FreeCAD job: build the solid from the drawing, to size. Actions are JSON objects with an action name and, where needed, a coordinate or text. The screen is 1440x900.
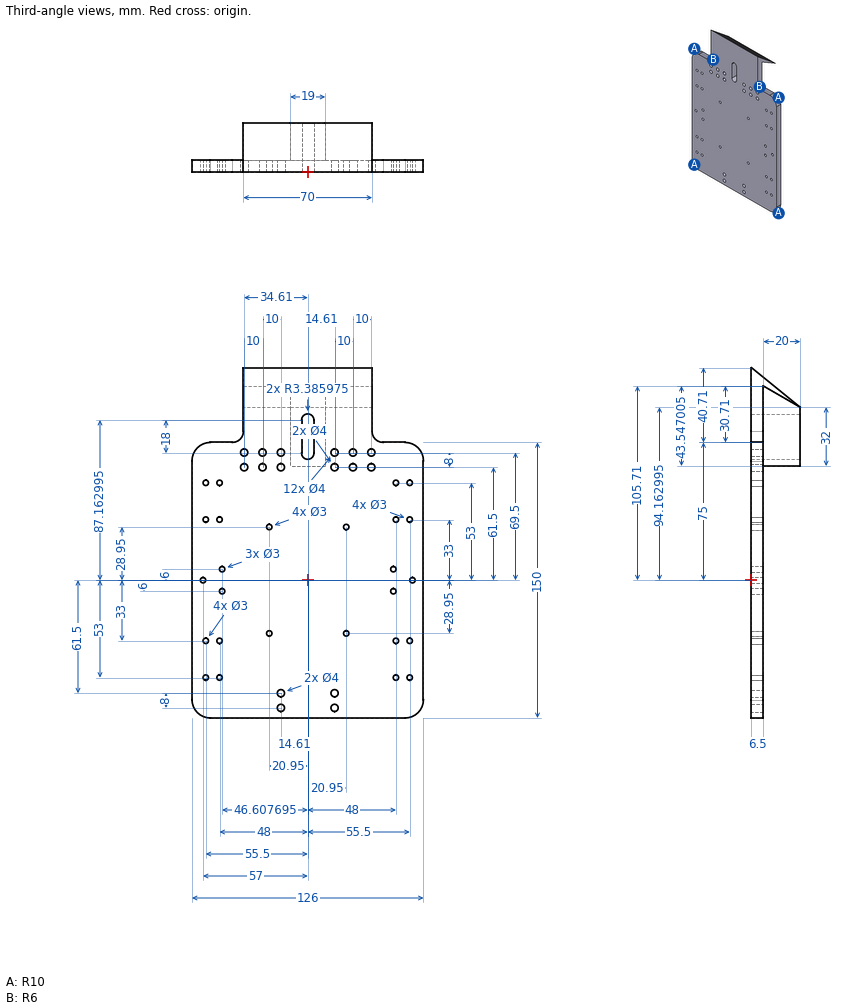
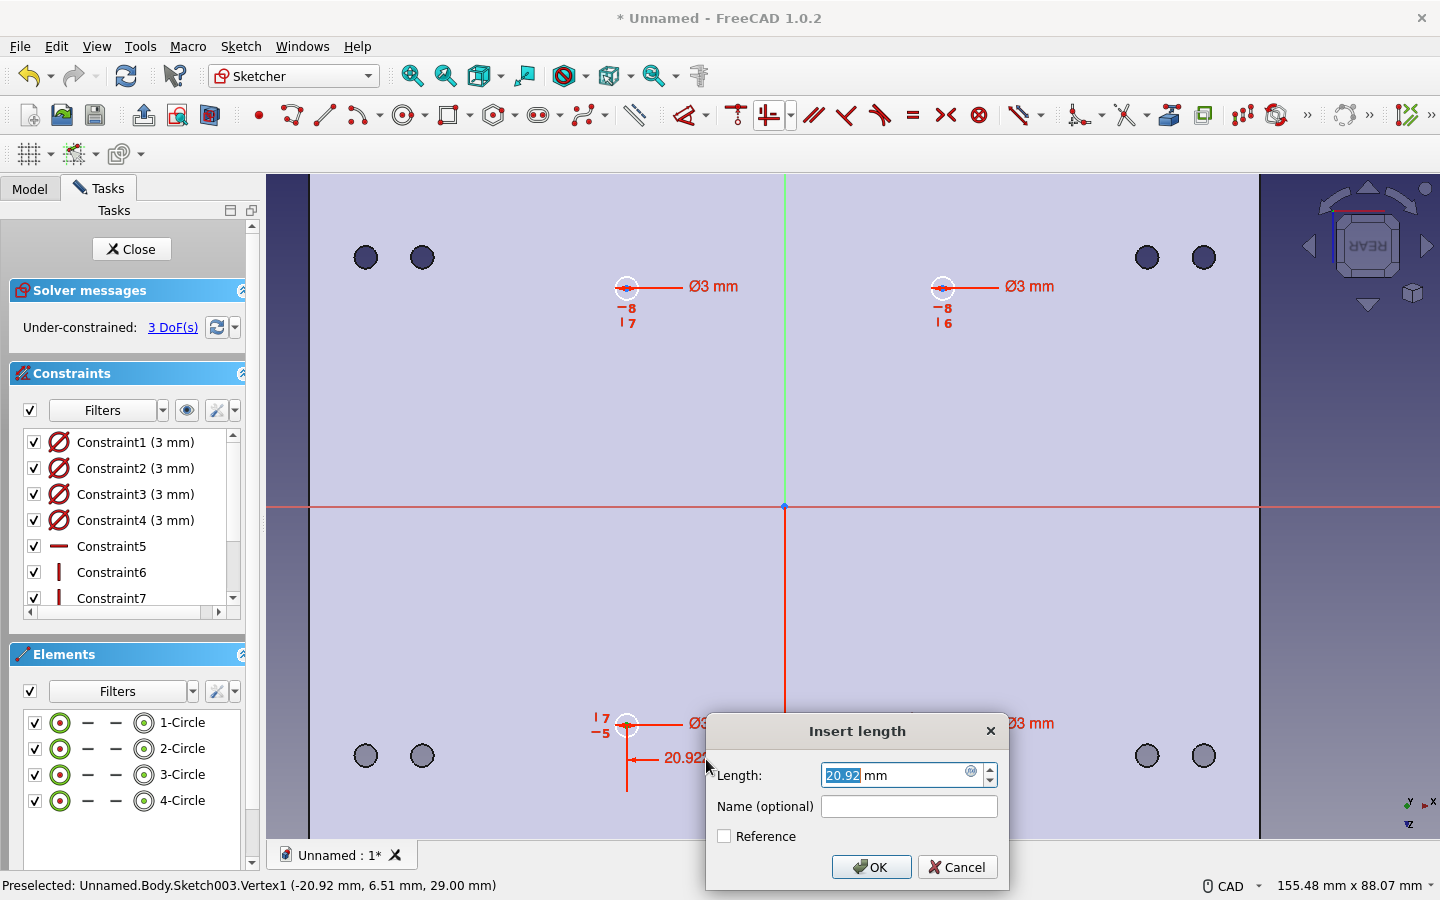
{"action": "type", "text": "20.95"}
{"action": "key", "text": "Return"}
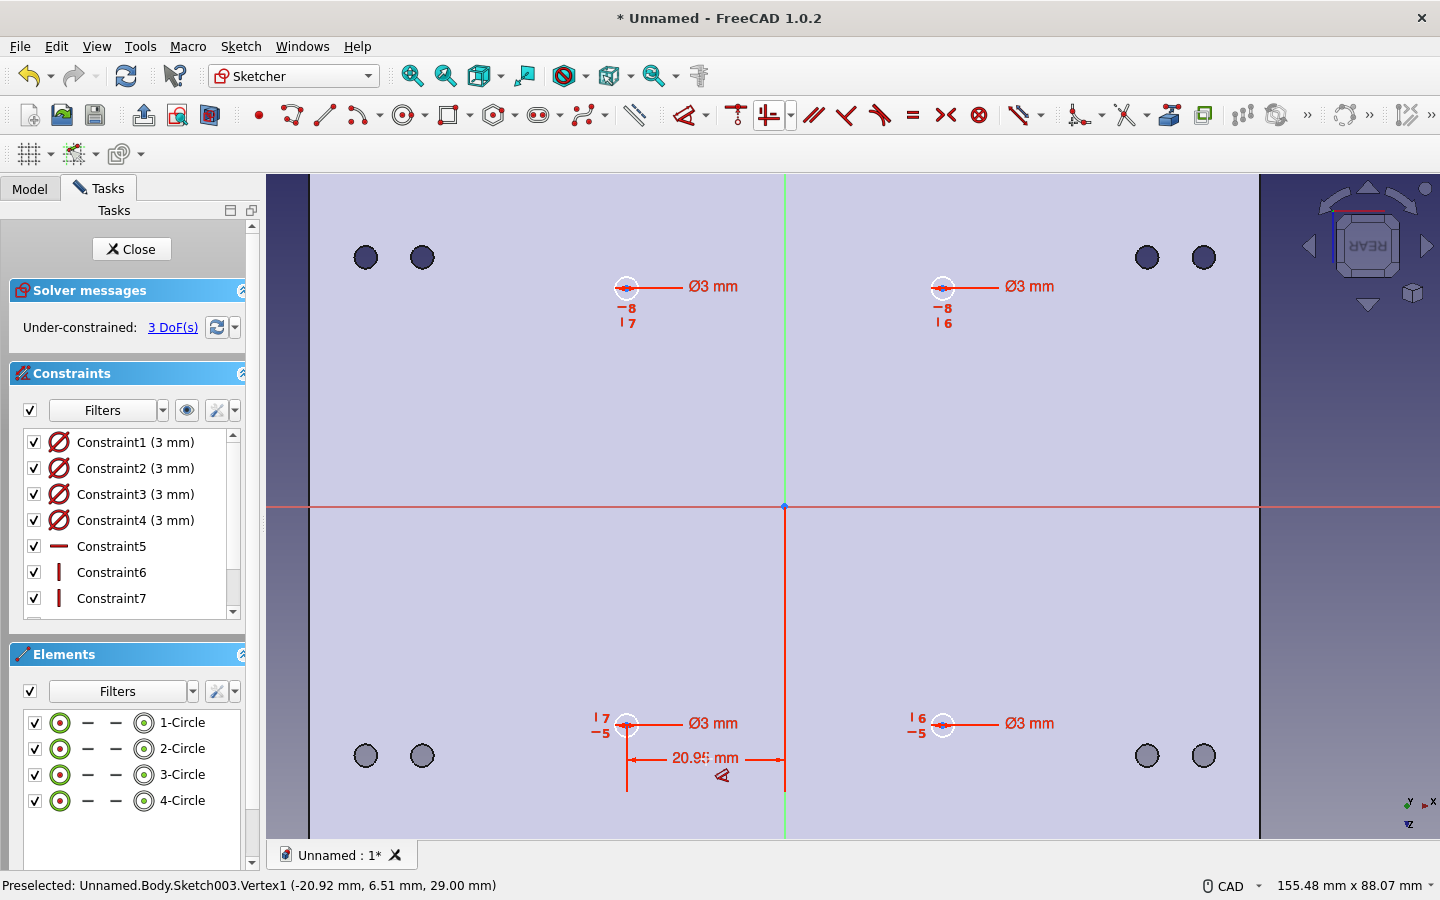
{"action": "left_click", "coordinate": [627, 725]}
{"action": "left_click", "coordinate": [593, 616]}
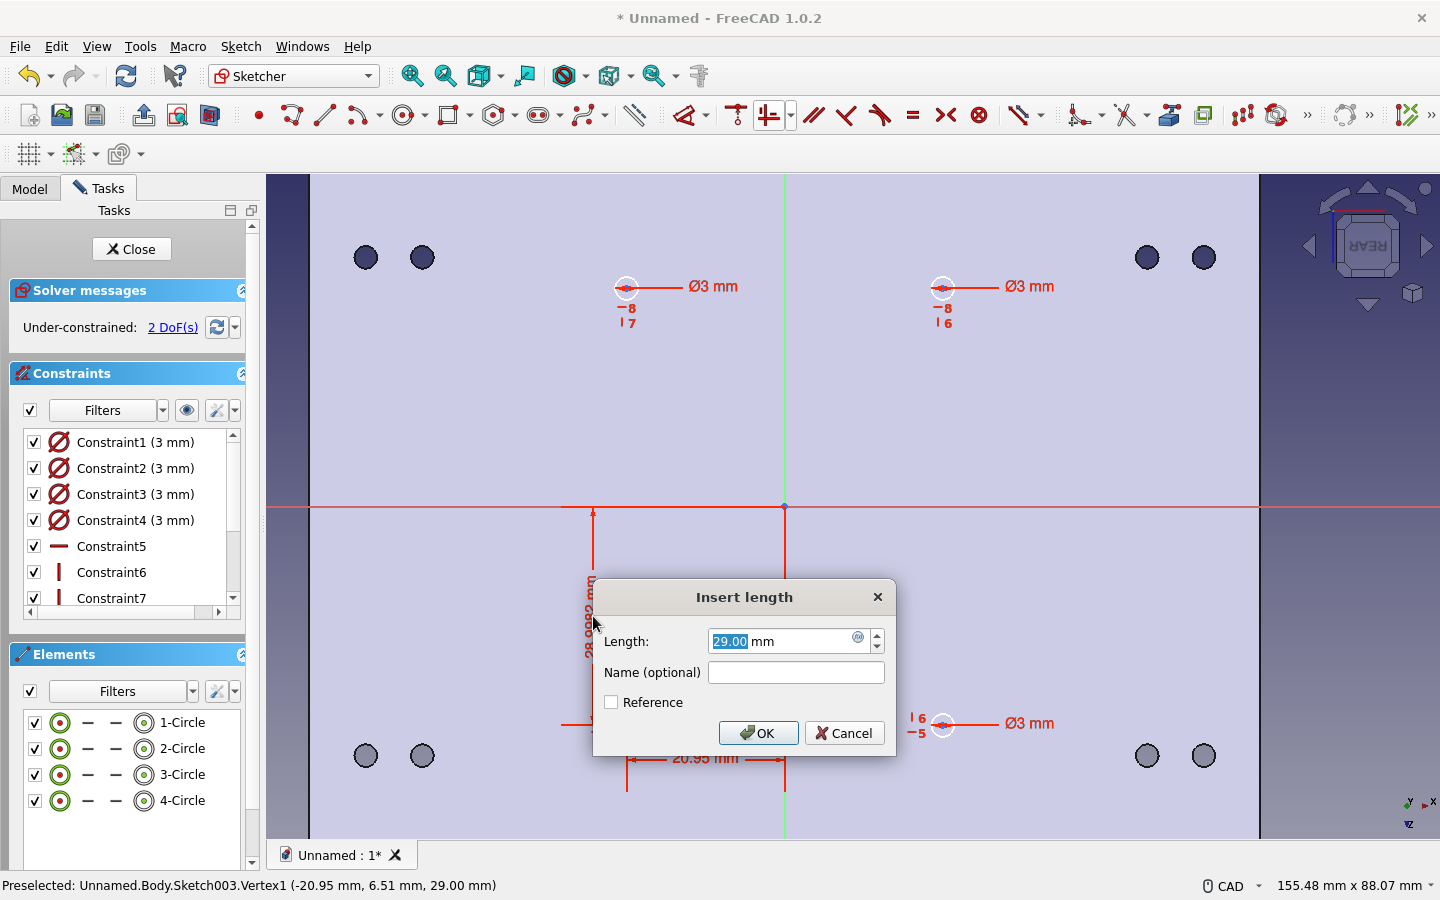
{"action": "type", "text": "28.95"}
{"action": "key", "text": "Return"}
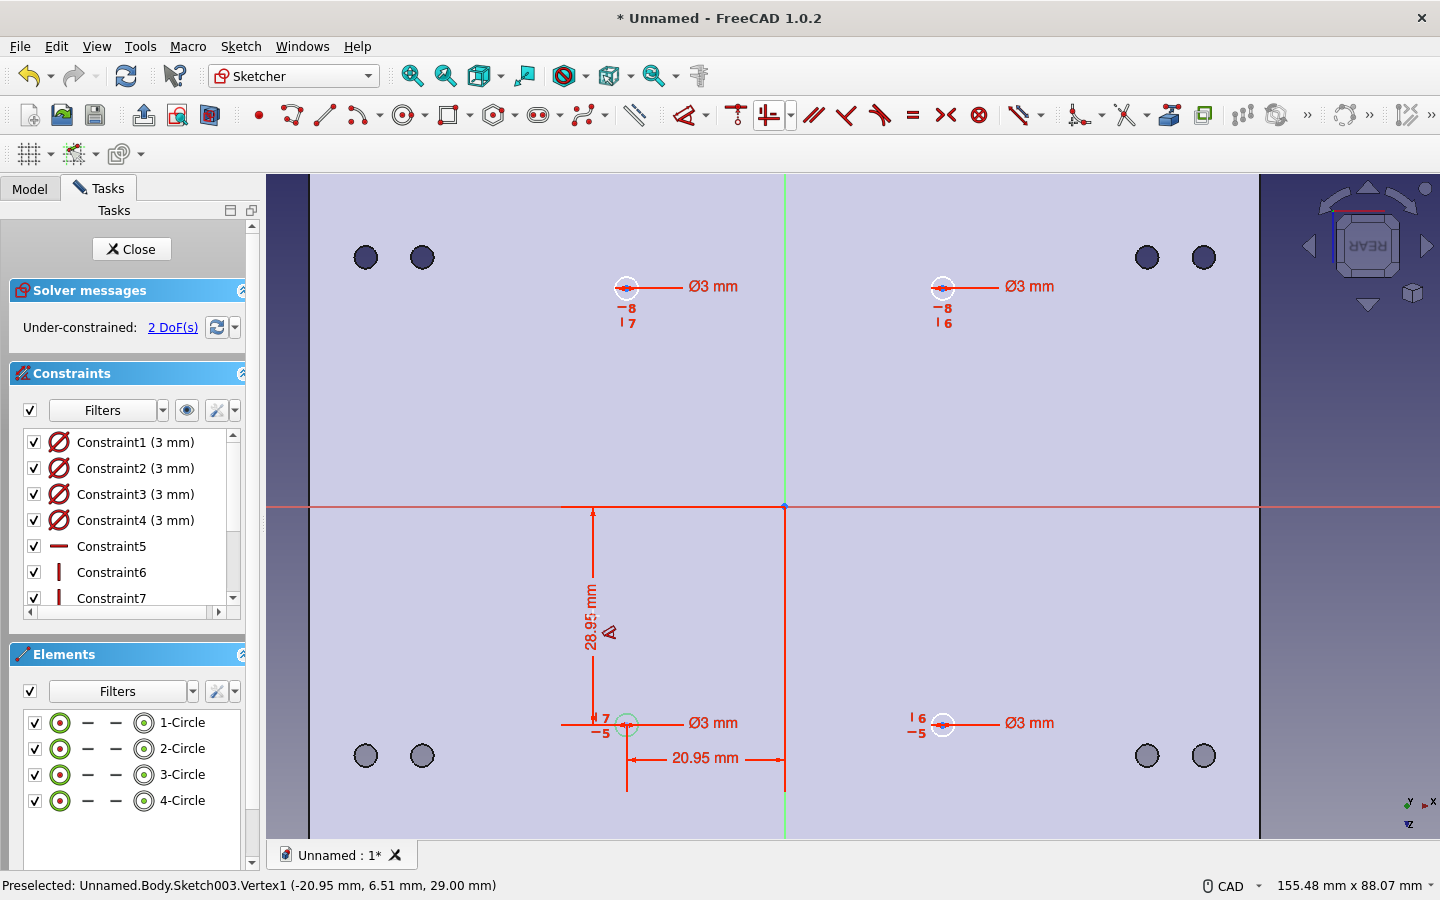
{"action": "left_click", "coordinate": [943, 725]}
{"action": "left_click", "coordinate": [864, 759]}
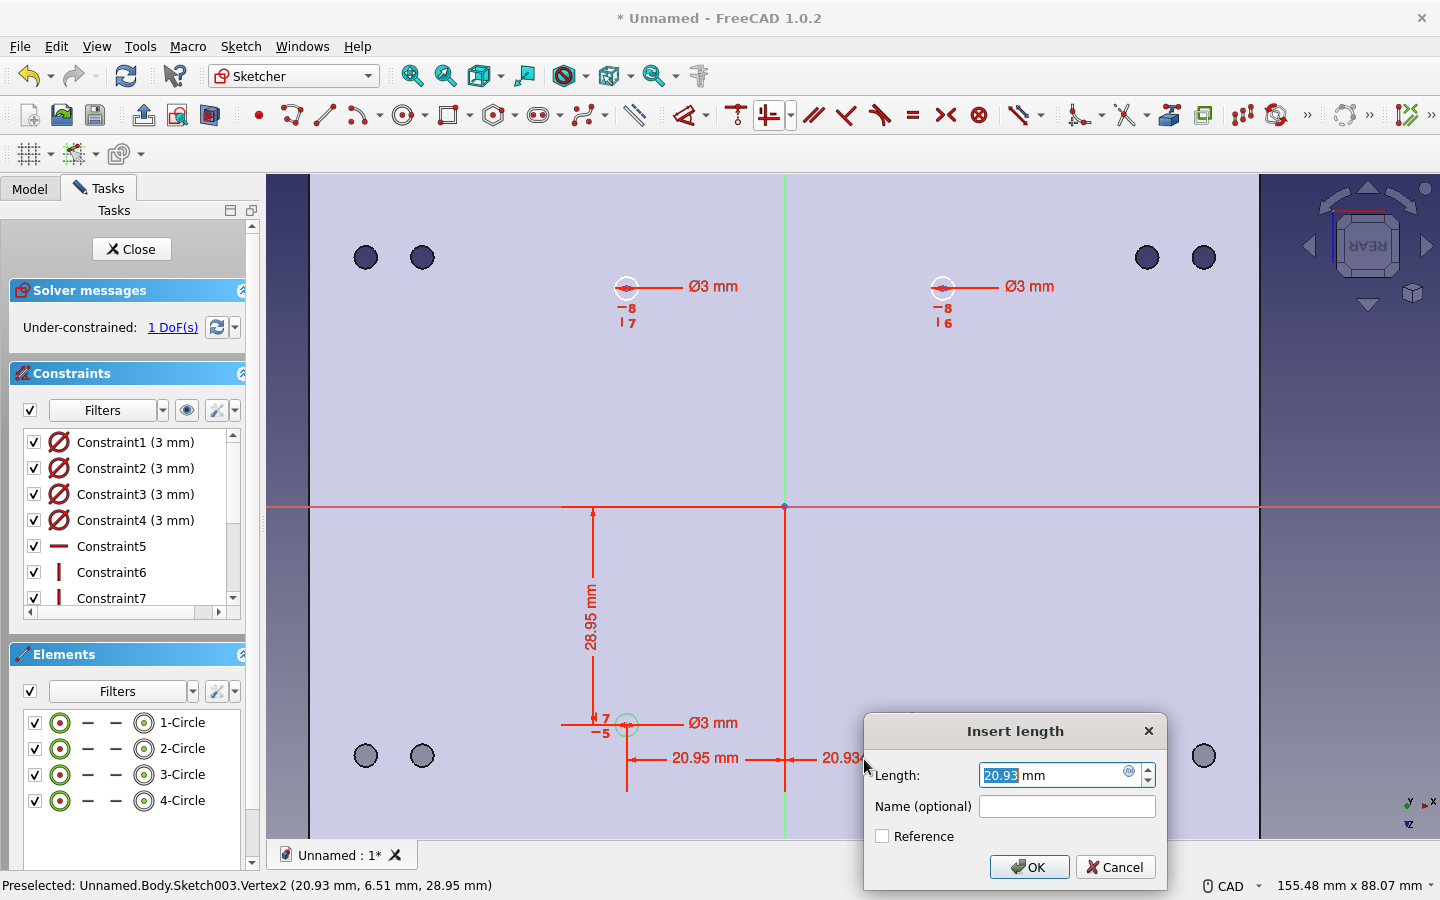
{"action": "type", "text": "20.95"}
{"action": "key", "text": "Return"}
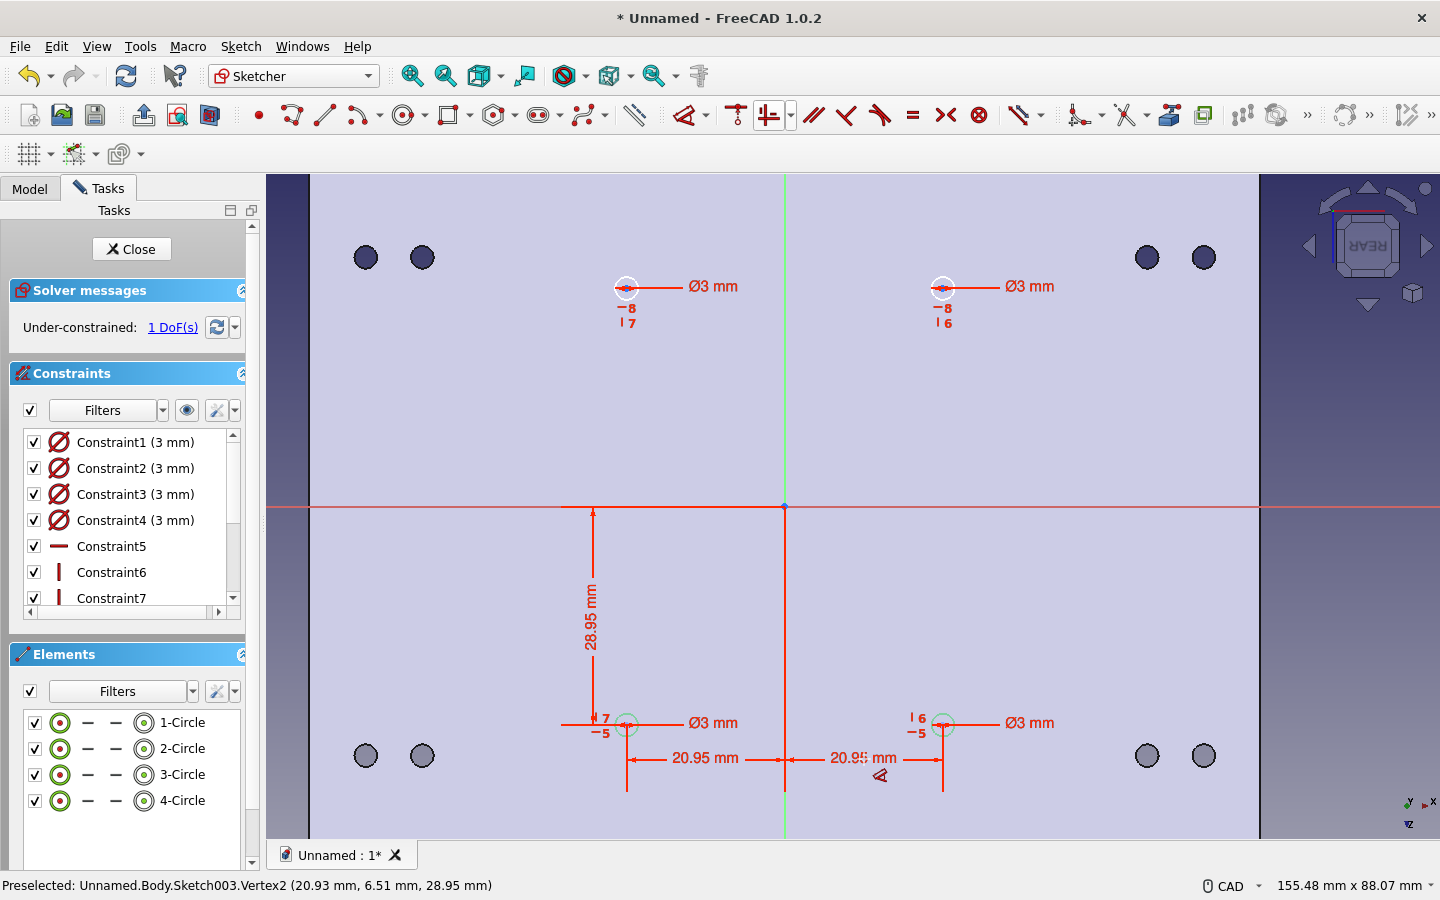
{"action": "left_click", "coordinate": [943, 288]}
{"action": "left_click", "coordinate": [977, 397]}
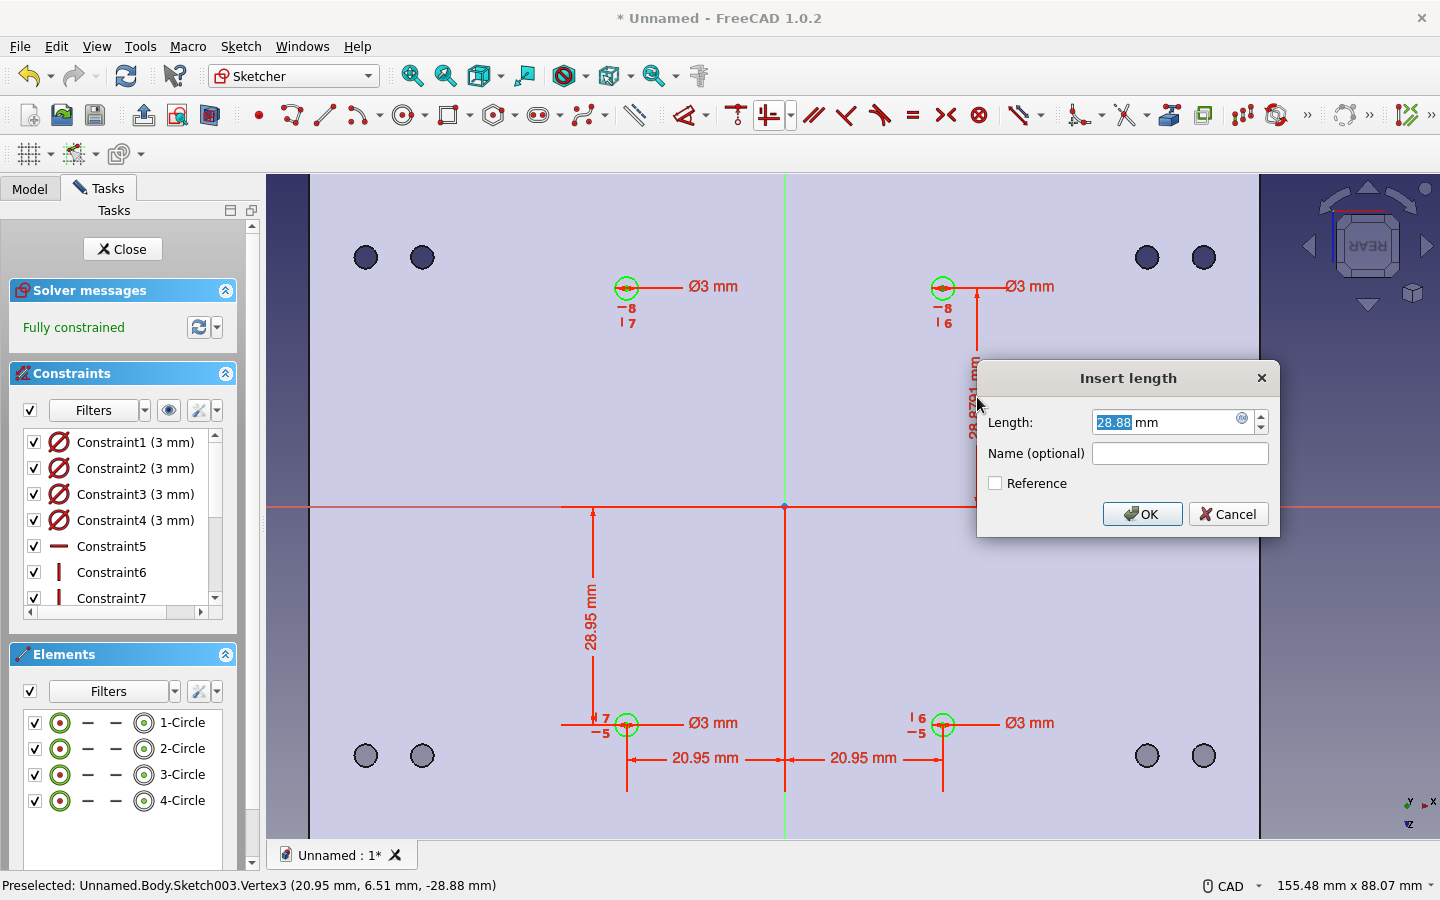
{"action": "type", "text": "28.95"}
{"action": "key", "text": "Return"}
{"action": "key", "text": "Escape"}